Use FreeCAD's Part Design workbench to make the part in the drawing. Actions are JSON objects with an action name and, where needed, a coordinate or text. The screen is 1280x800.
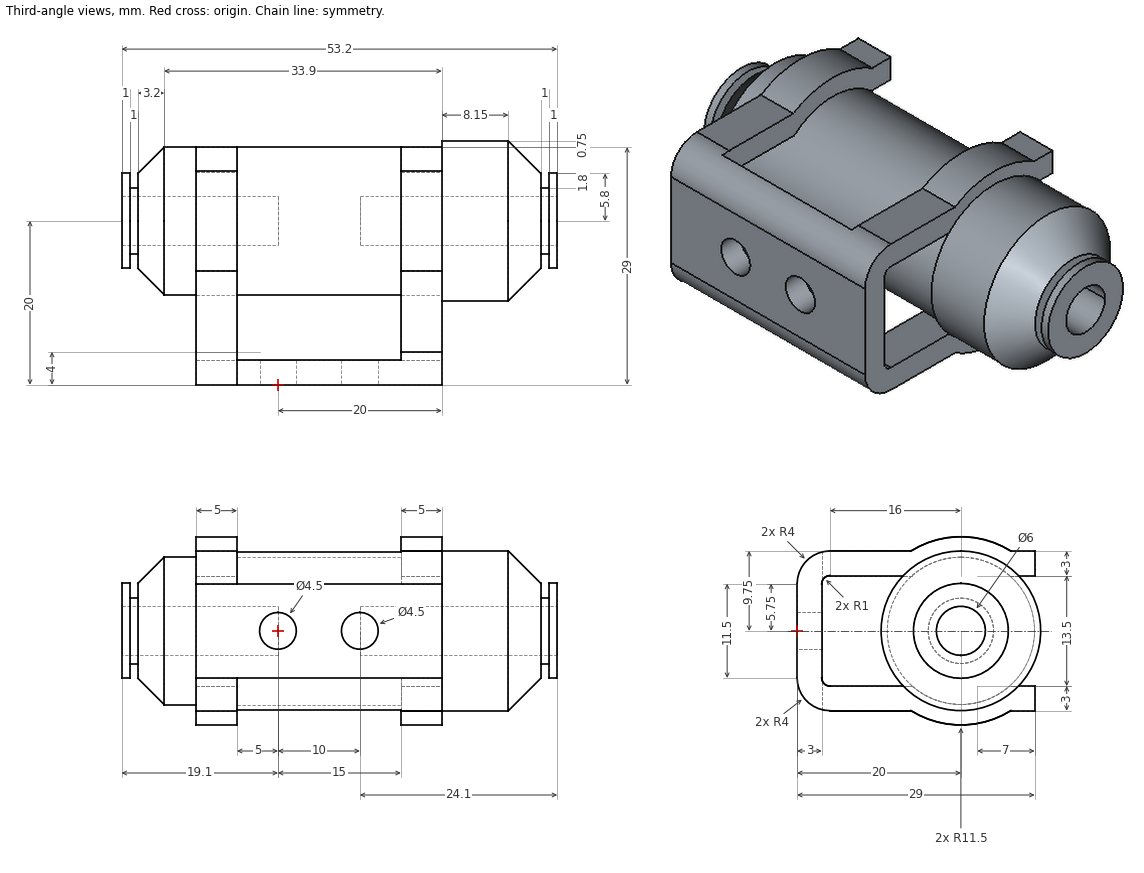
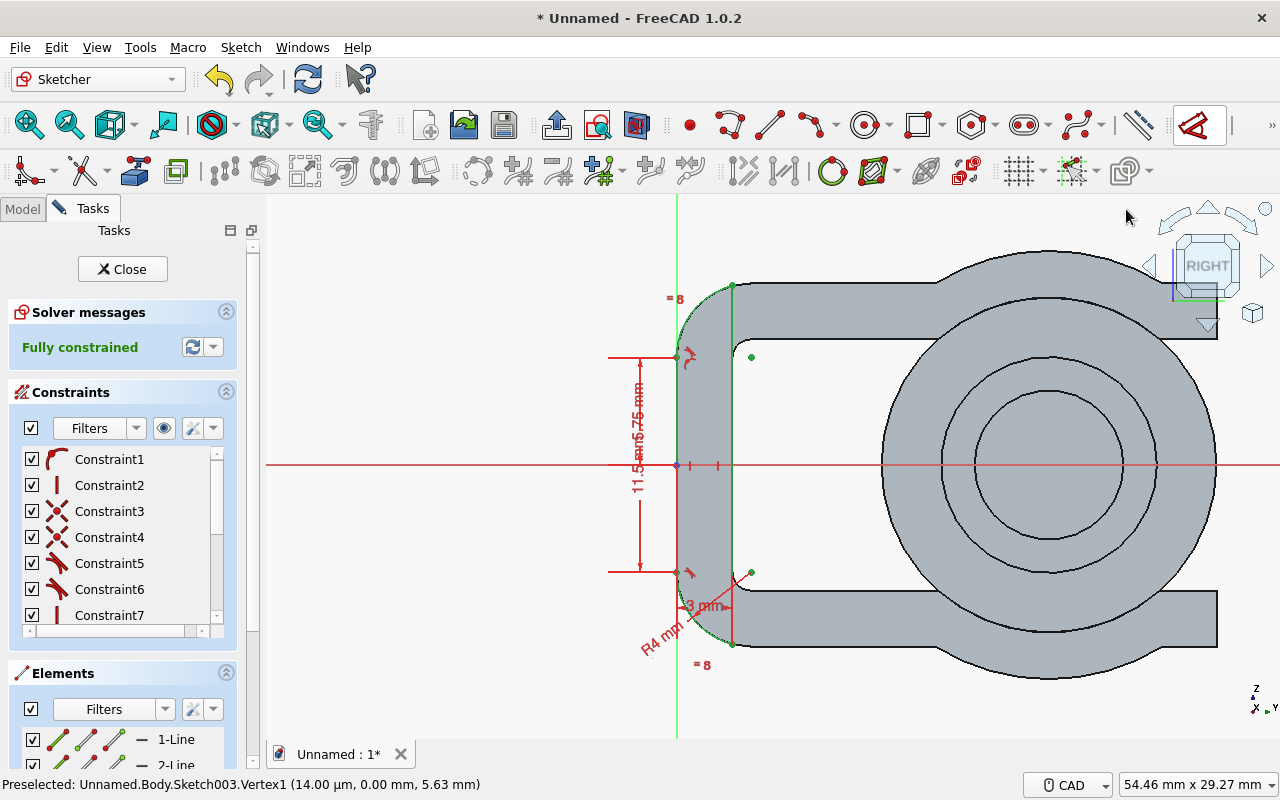
{"action": "left_click", "coordinate": [123, 269]}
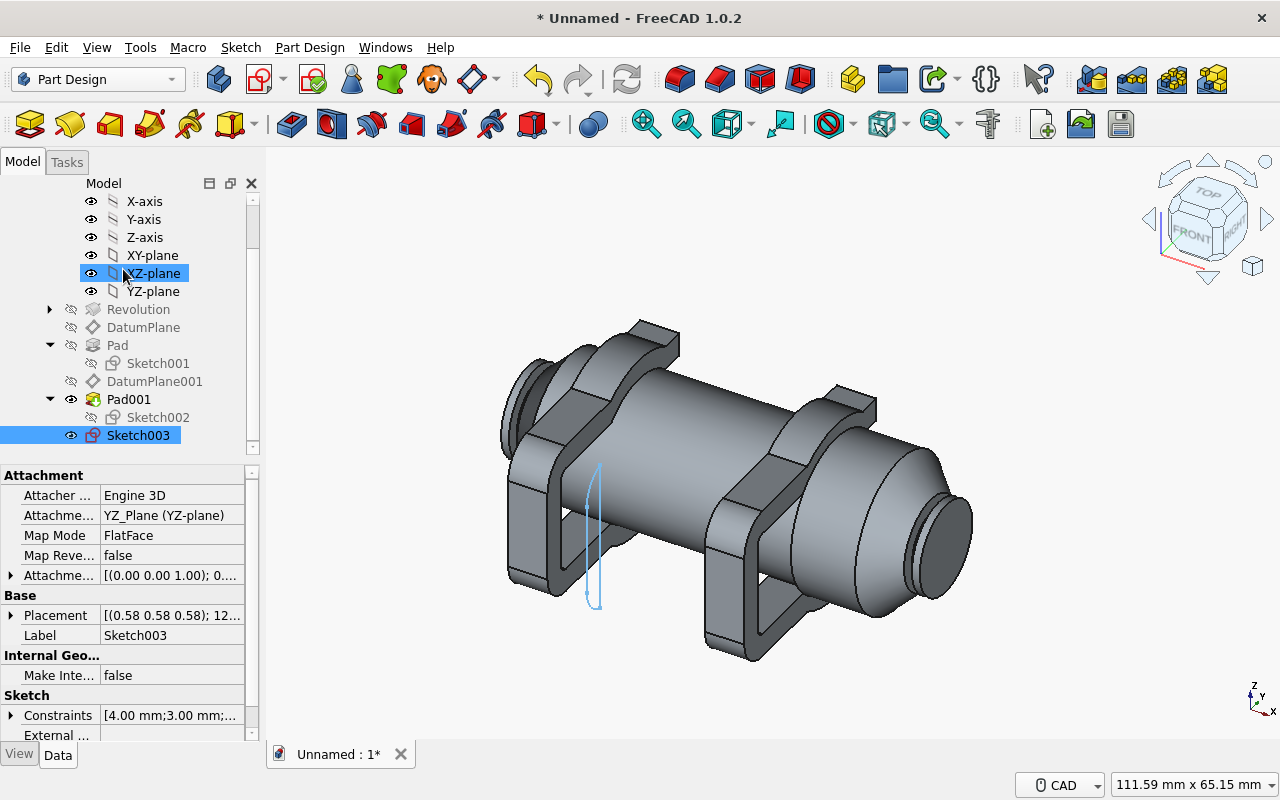
{"action": "left_click", "coordinate": [30, 124]}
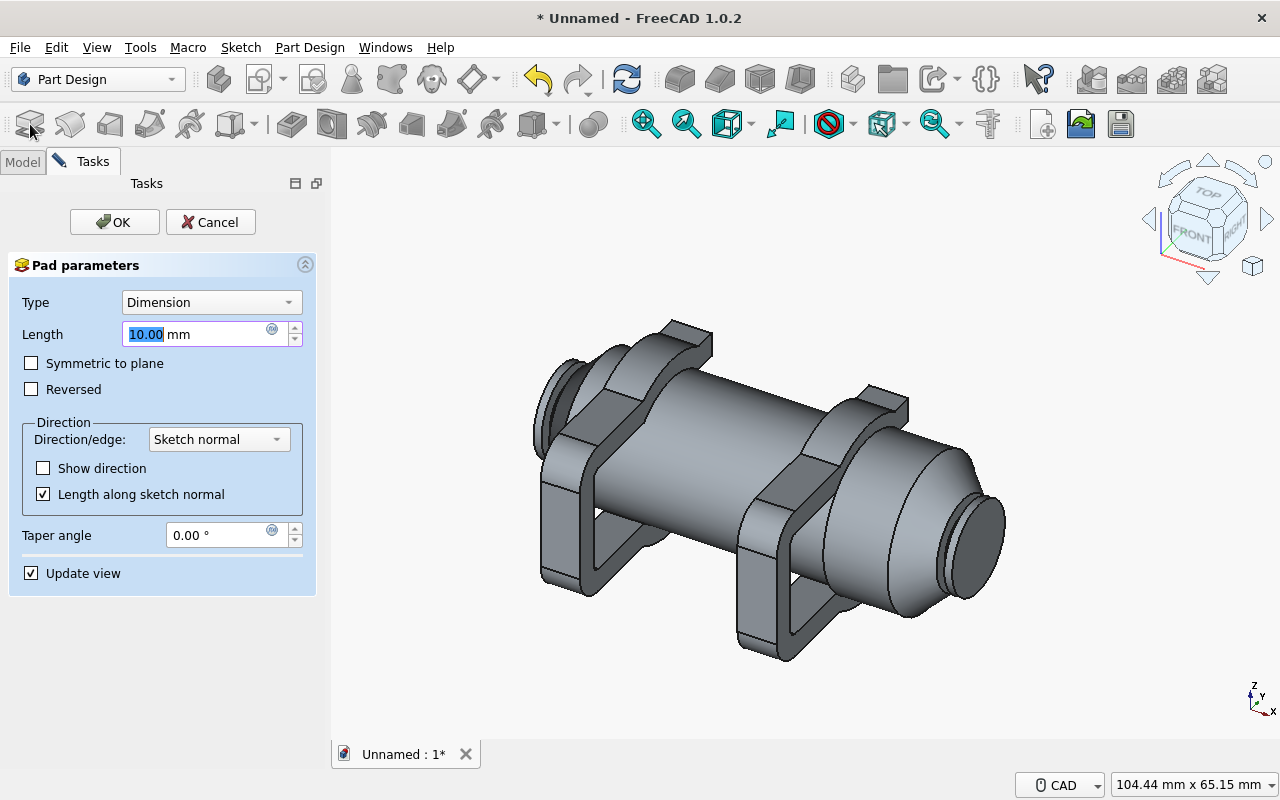
{"action": "type", "text": "15"}
{"action": "key", "text": "Tab"}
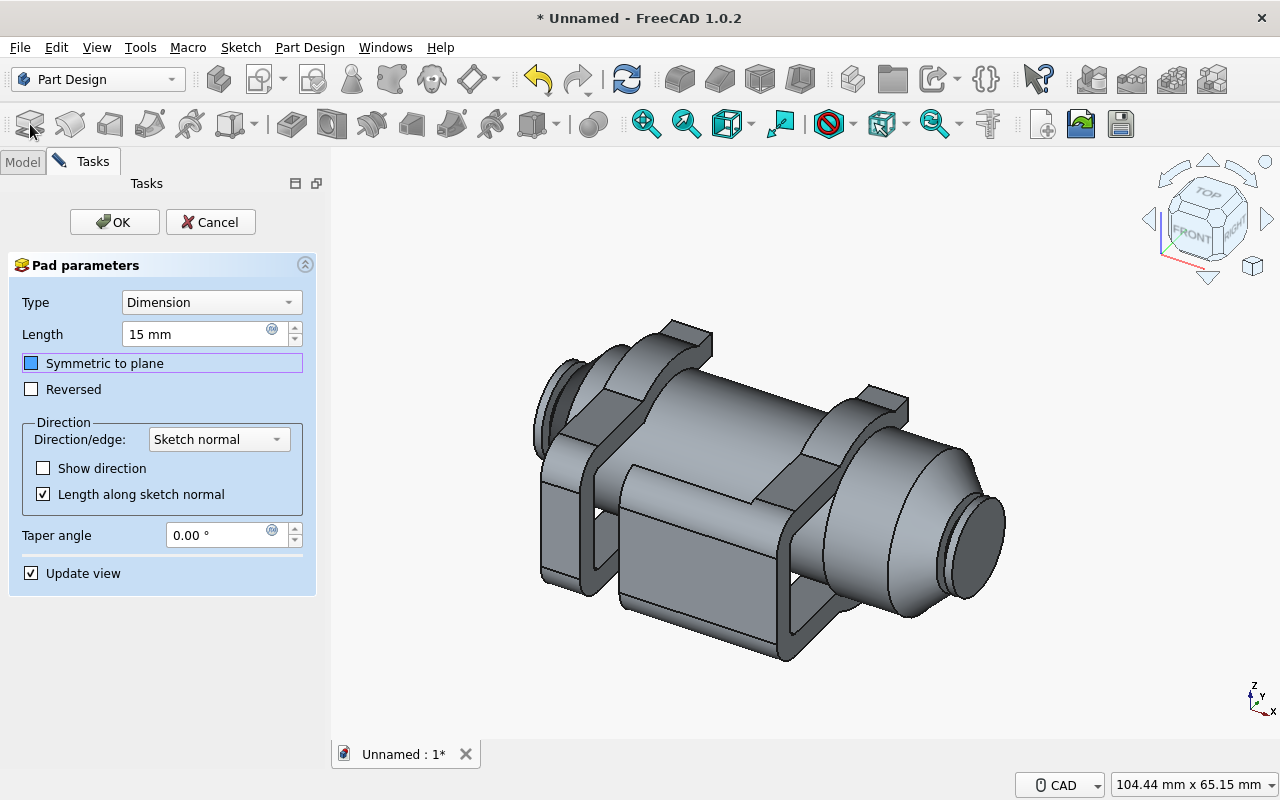
{"action": "left_click", "coordinate": [115, 222]}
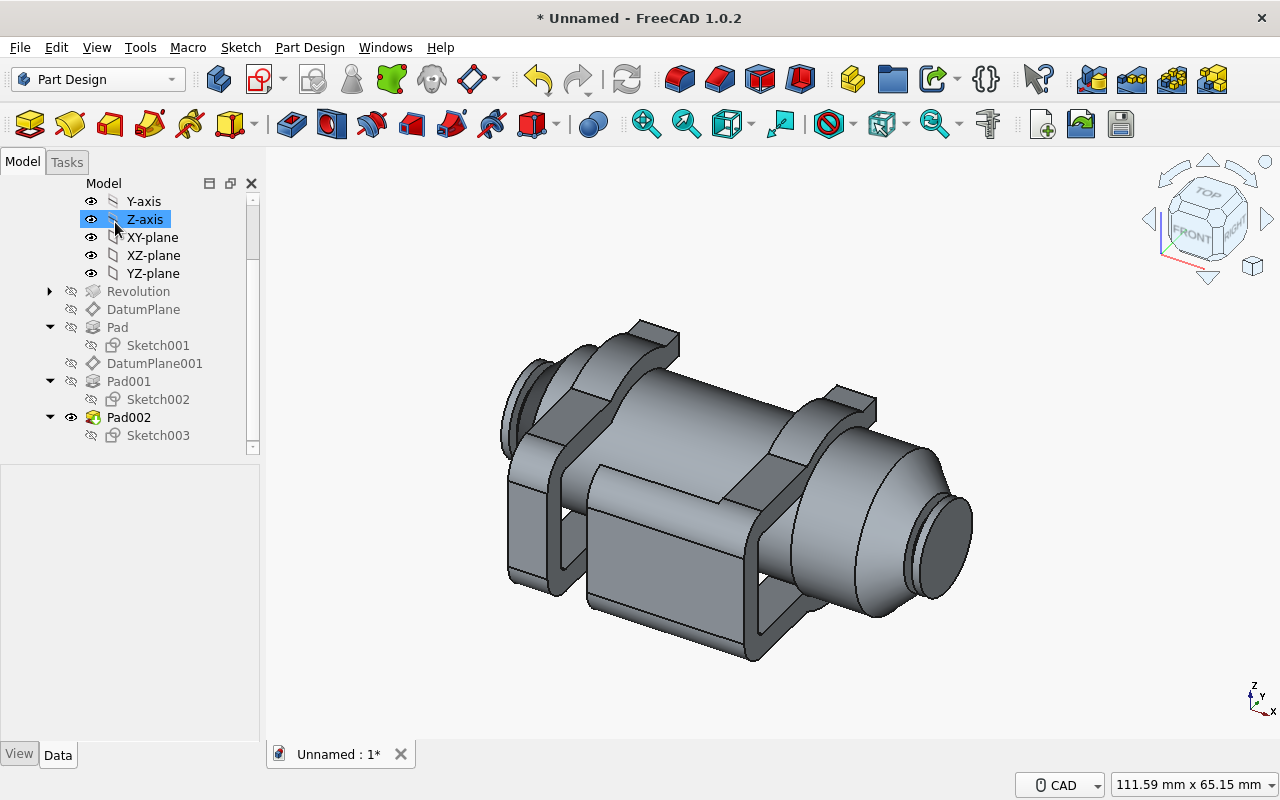
{"action": "scroll", "coordinate": [160, 323], "scroll_direction": "down", "scroll_amount": 3}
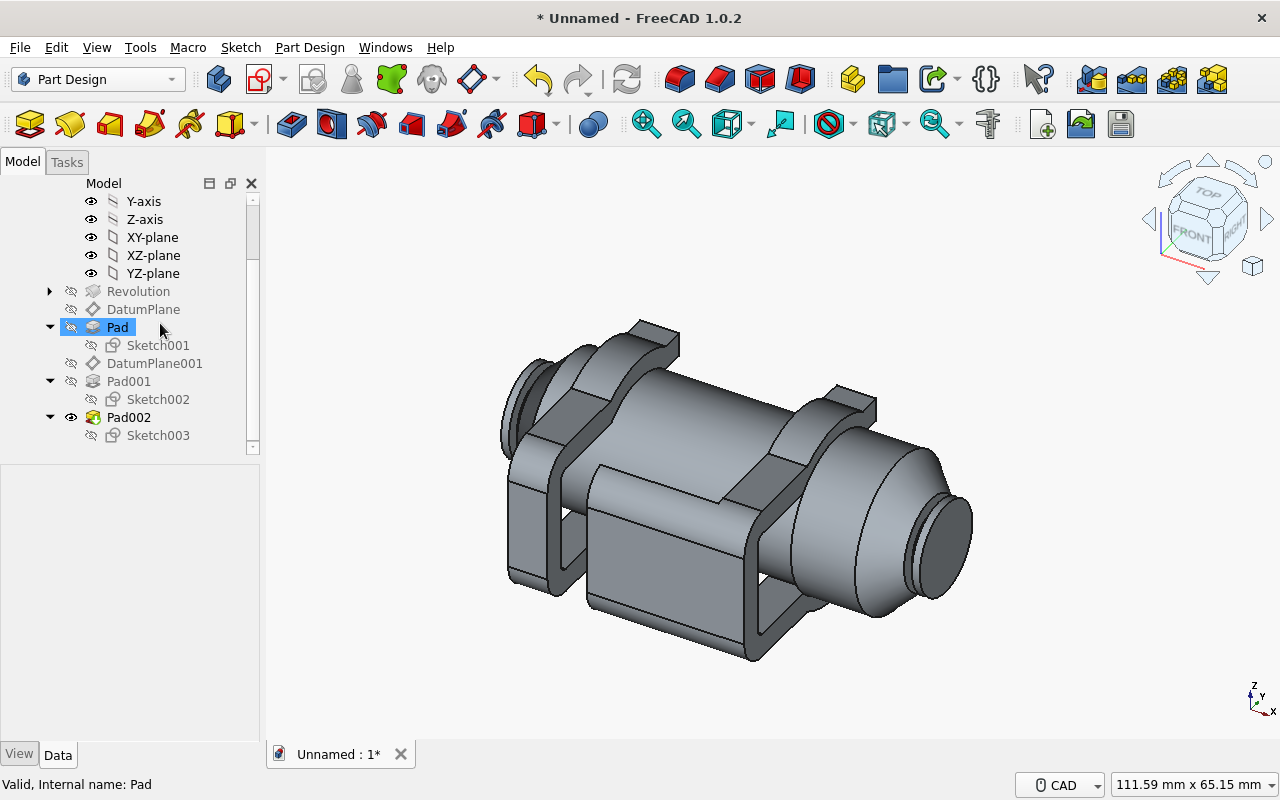
{"action": "scroll", "coordinate": [160, 323], "scroll_direction": "up", "scroll_amount": 15}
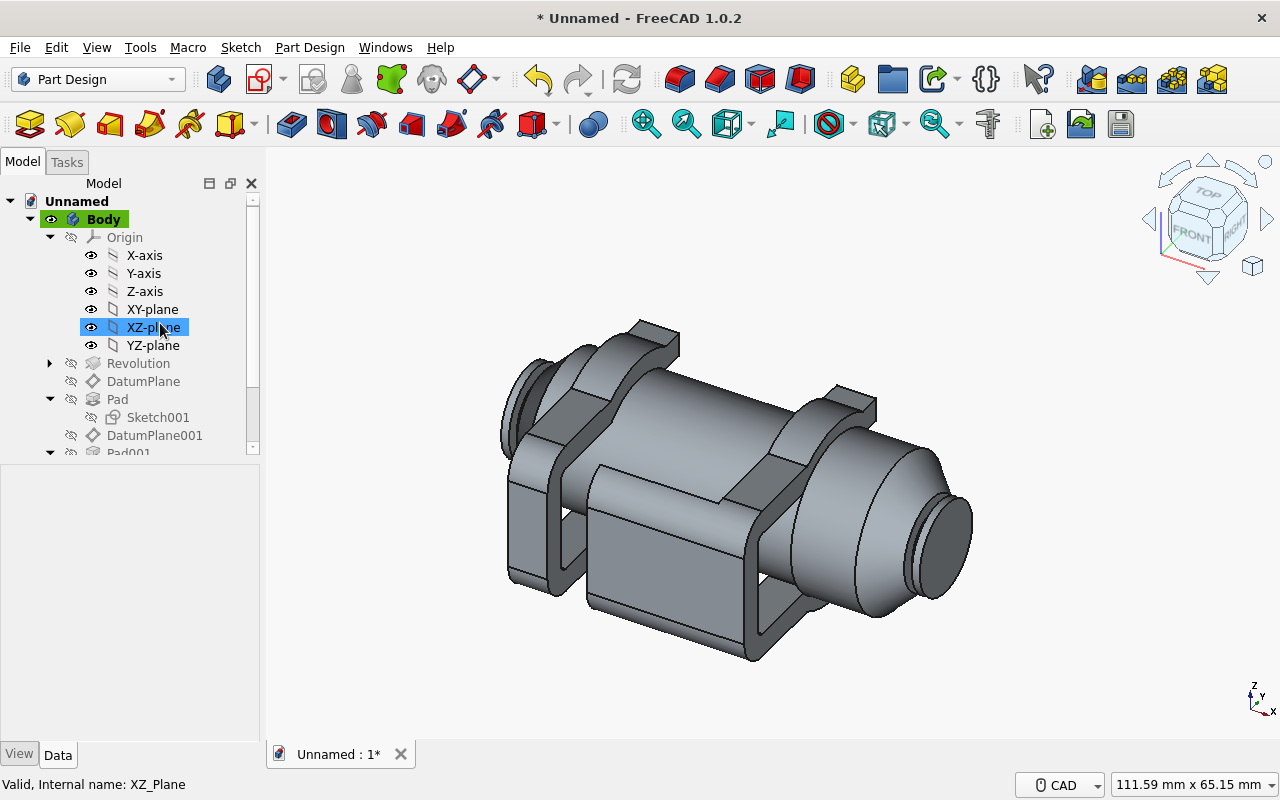
{"action": "left_click", "coordinate": [136, 345]}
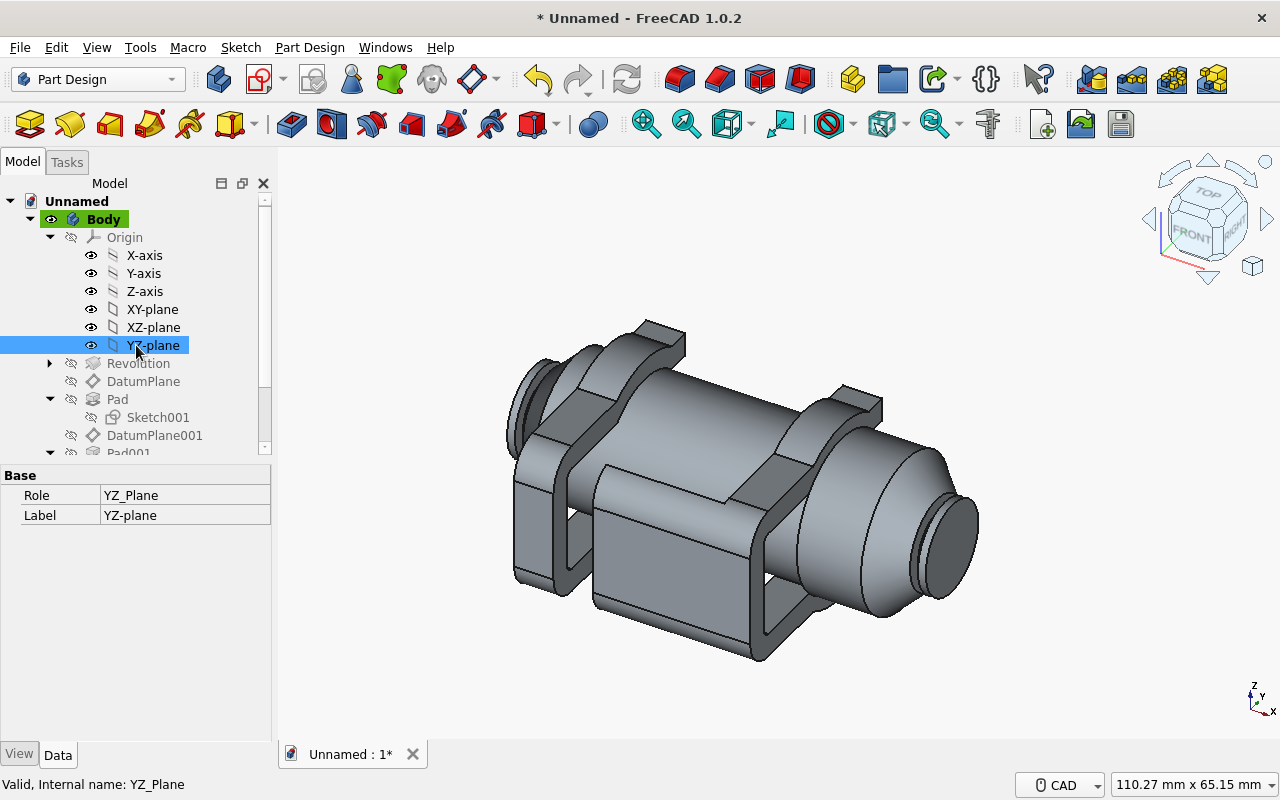
{"action": "left_click", "coordinate": [472, 80]}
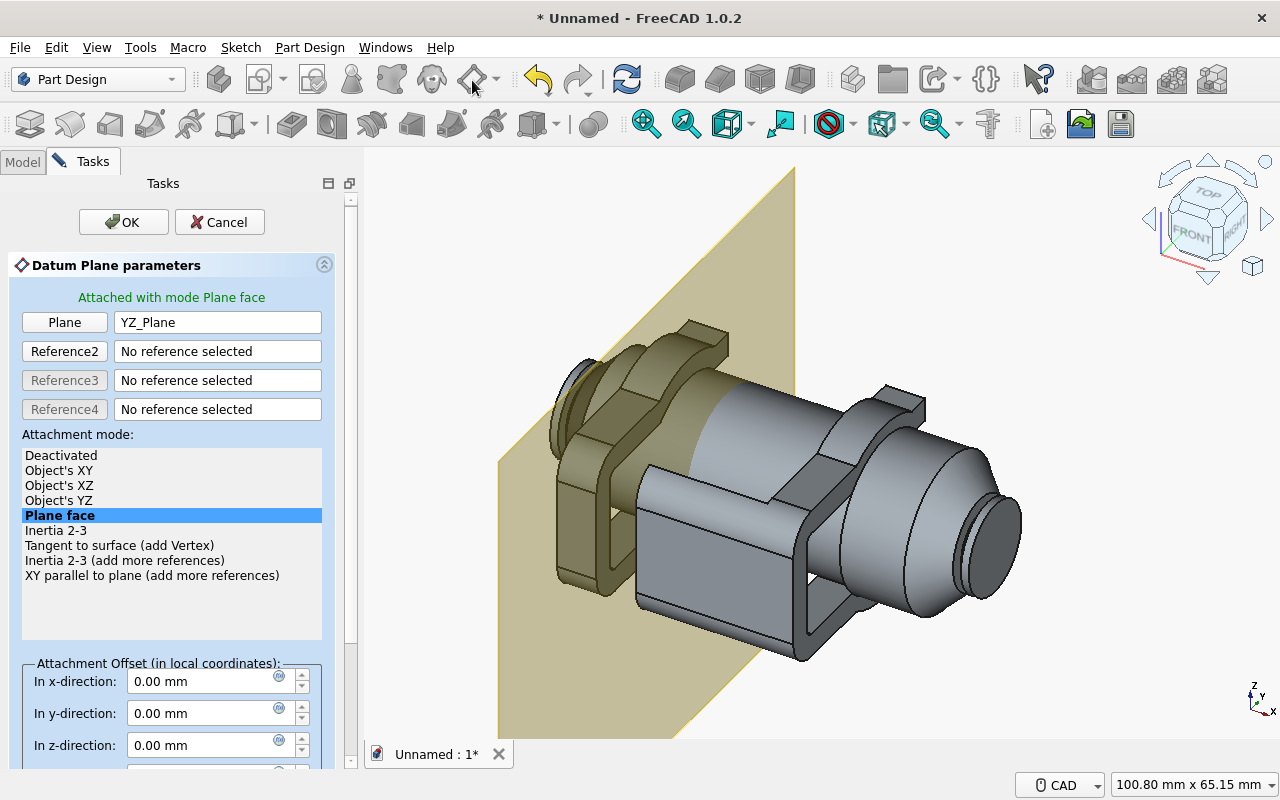
{"action": "triple_click", "coordinate": [210, 745]}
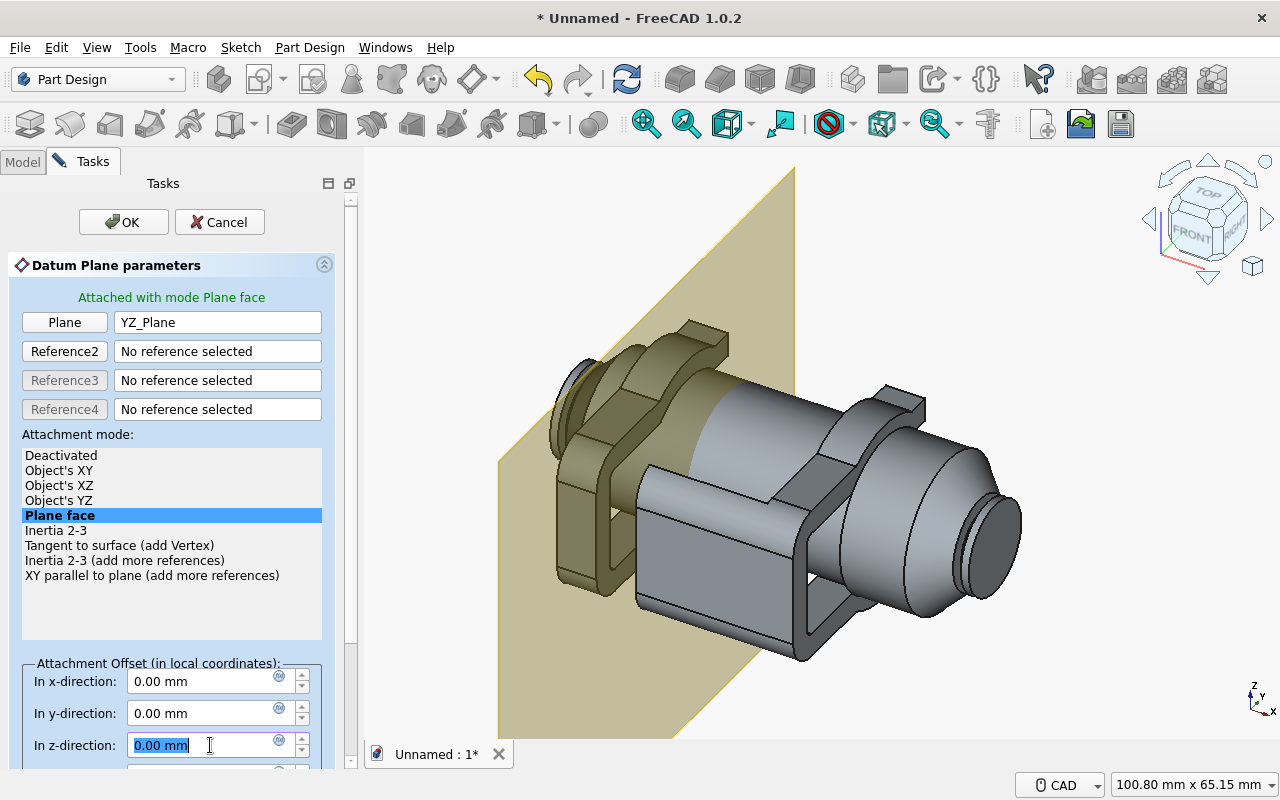
{"action": "type", "text": "-5"}
{"action": "key", "text": "Tab"}